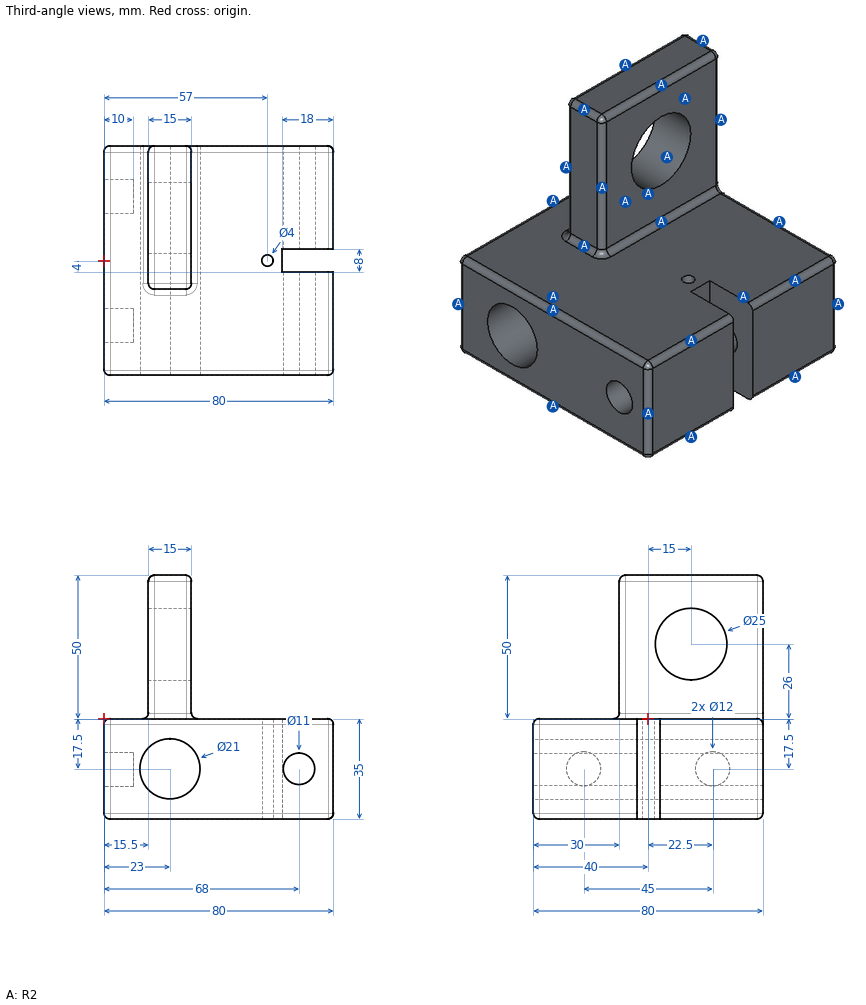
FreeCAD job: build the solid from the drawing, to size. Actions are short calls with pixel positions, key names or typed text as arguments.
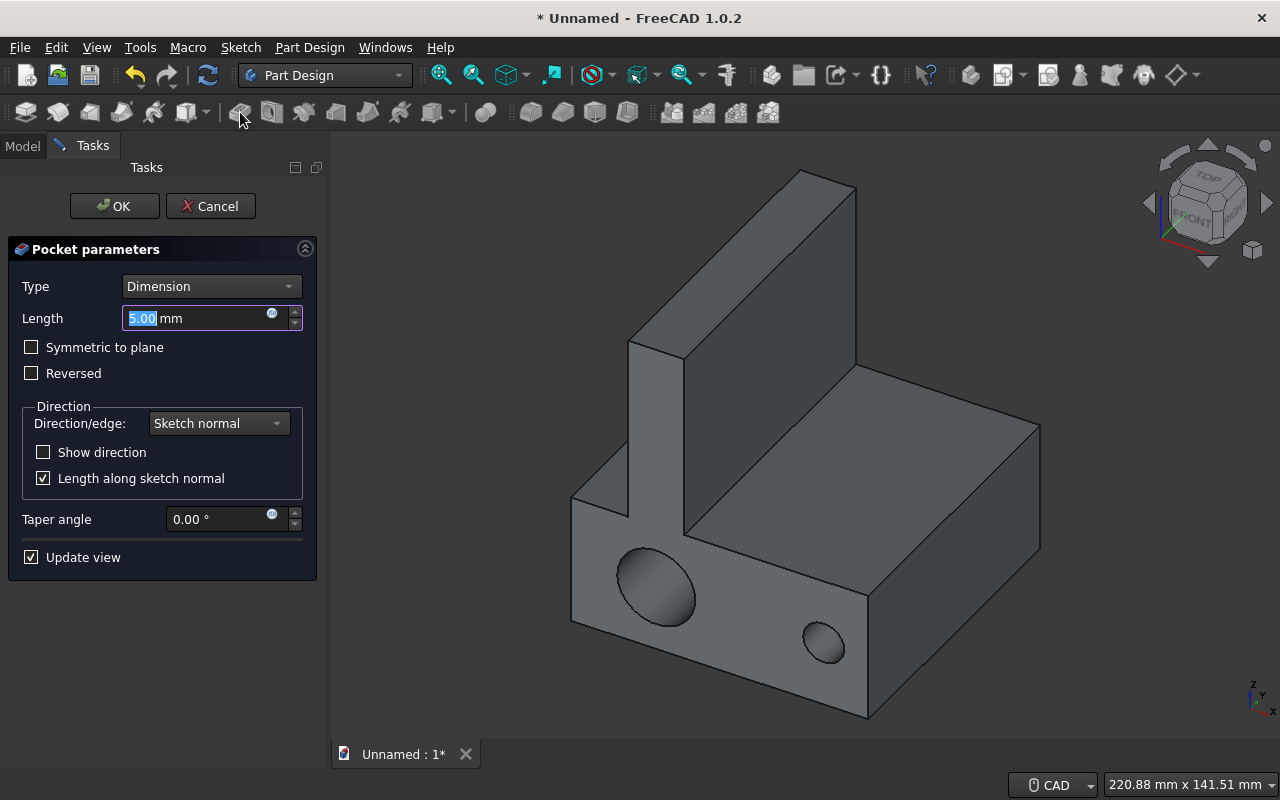
text(10)
key(Tab)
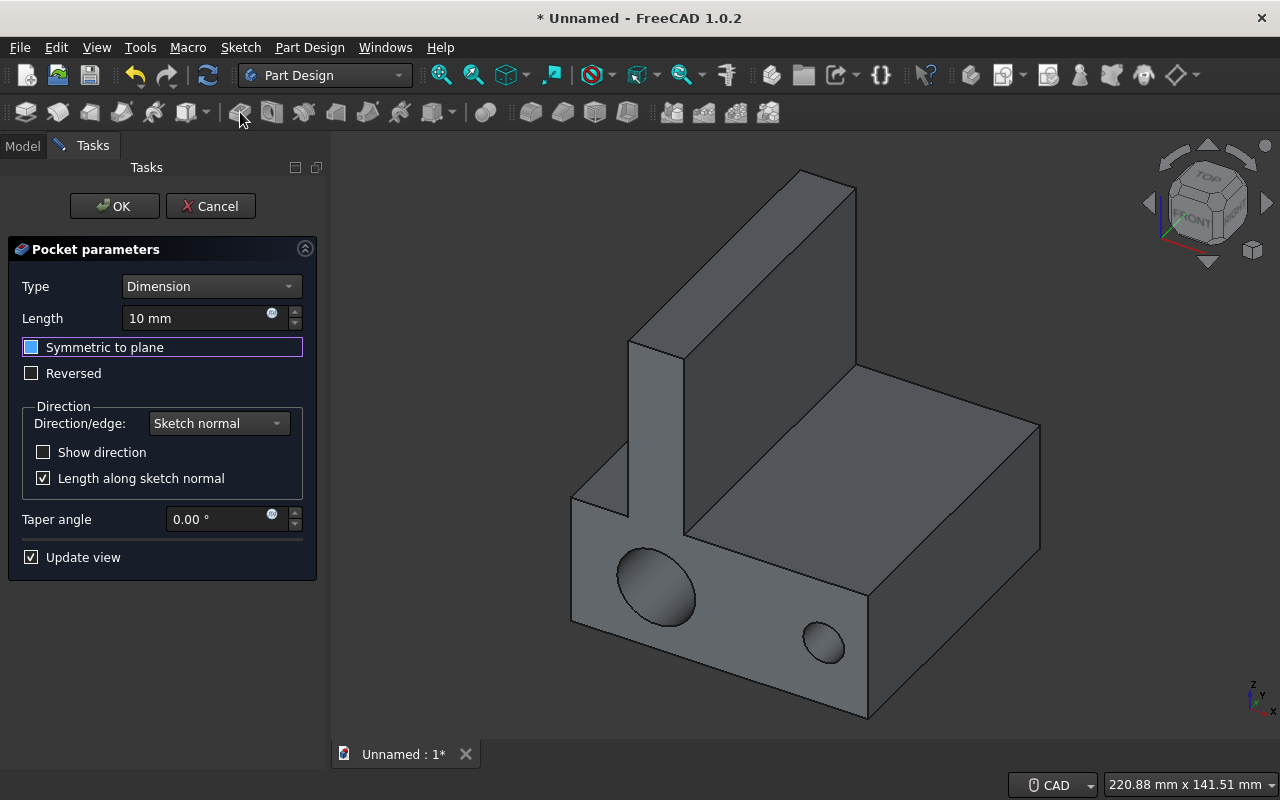
click(30, 373)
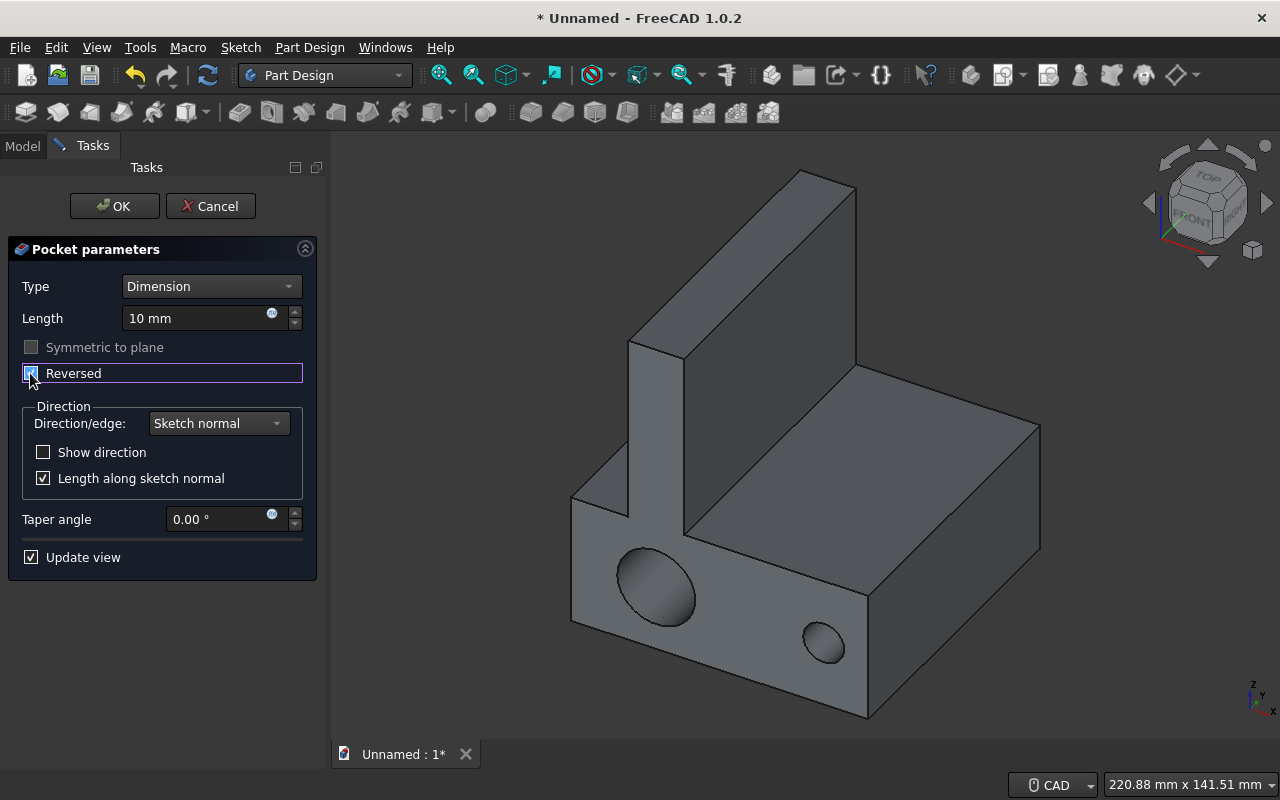
click(115, 206)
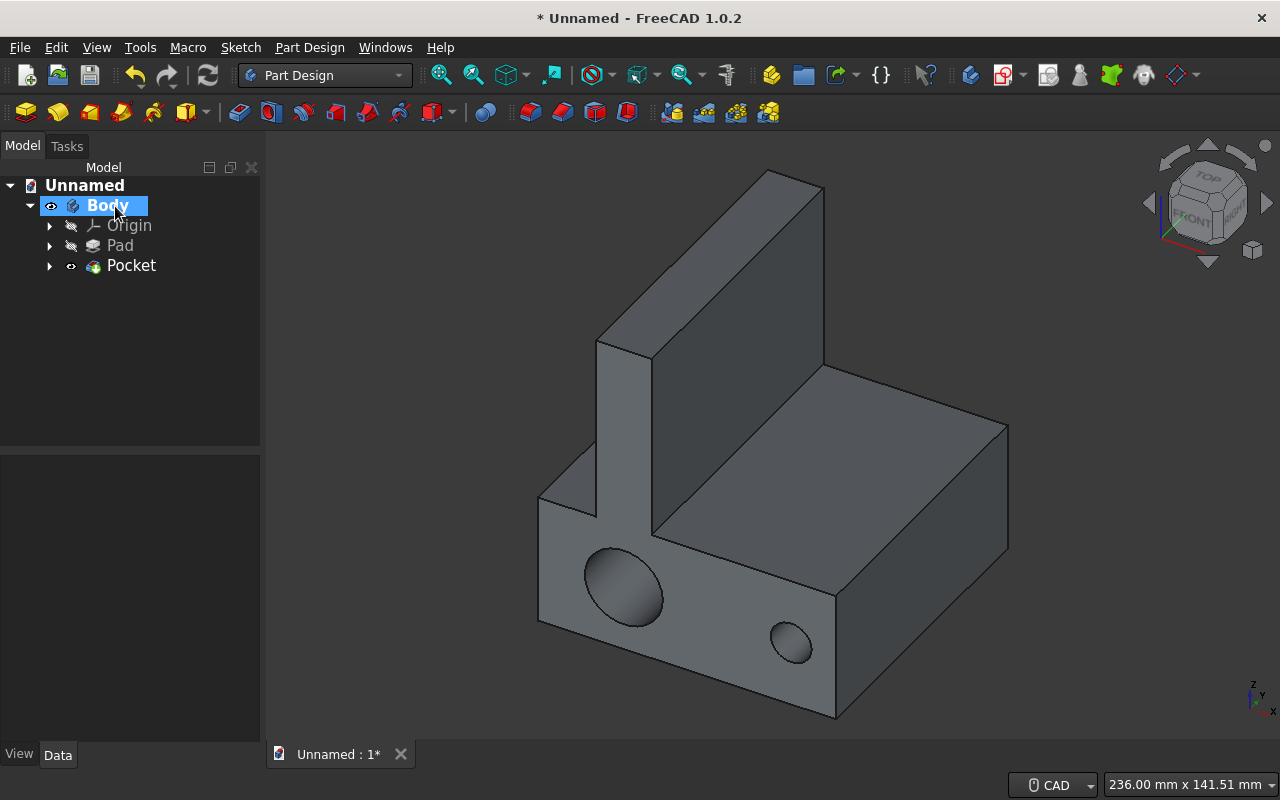
click(762, 336)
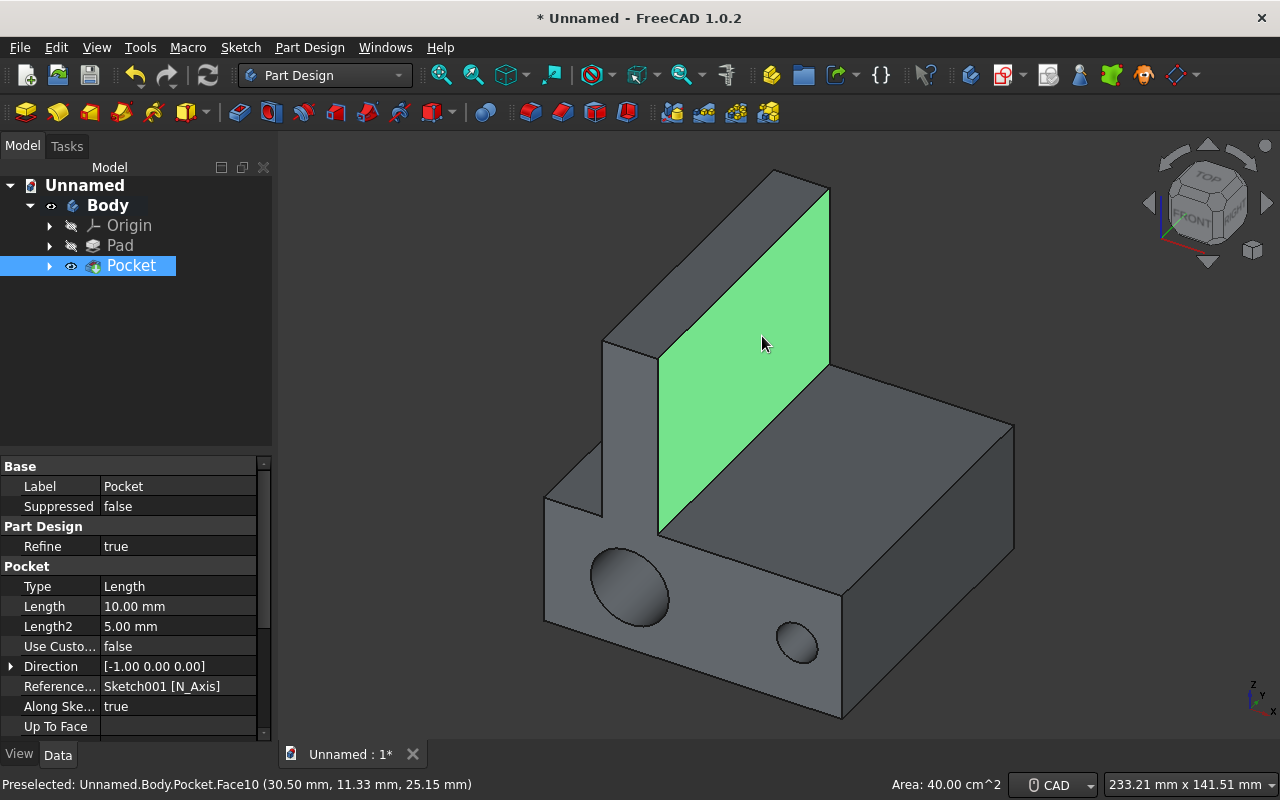
click(1004, 76)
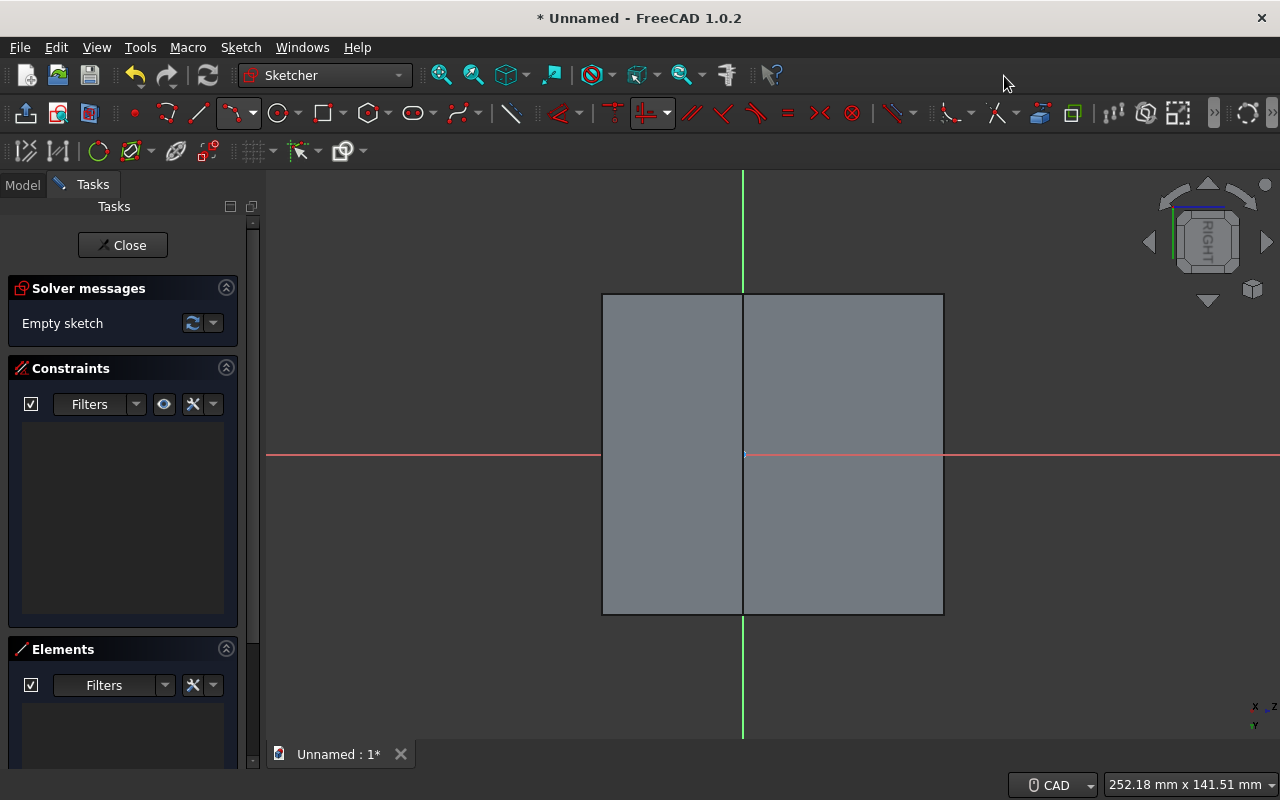
scroll(957, 308, up, 4)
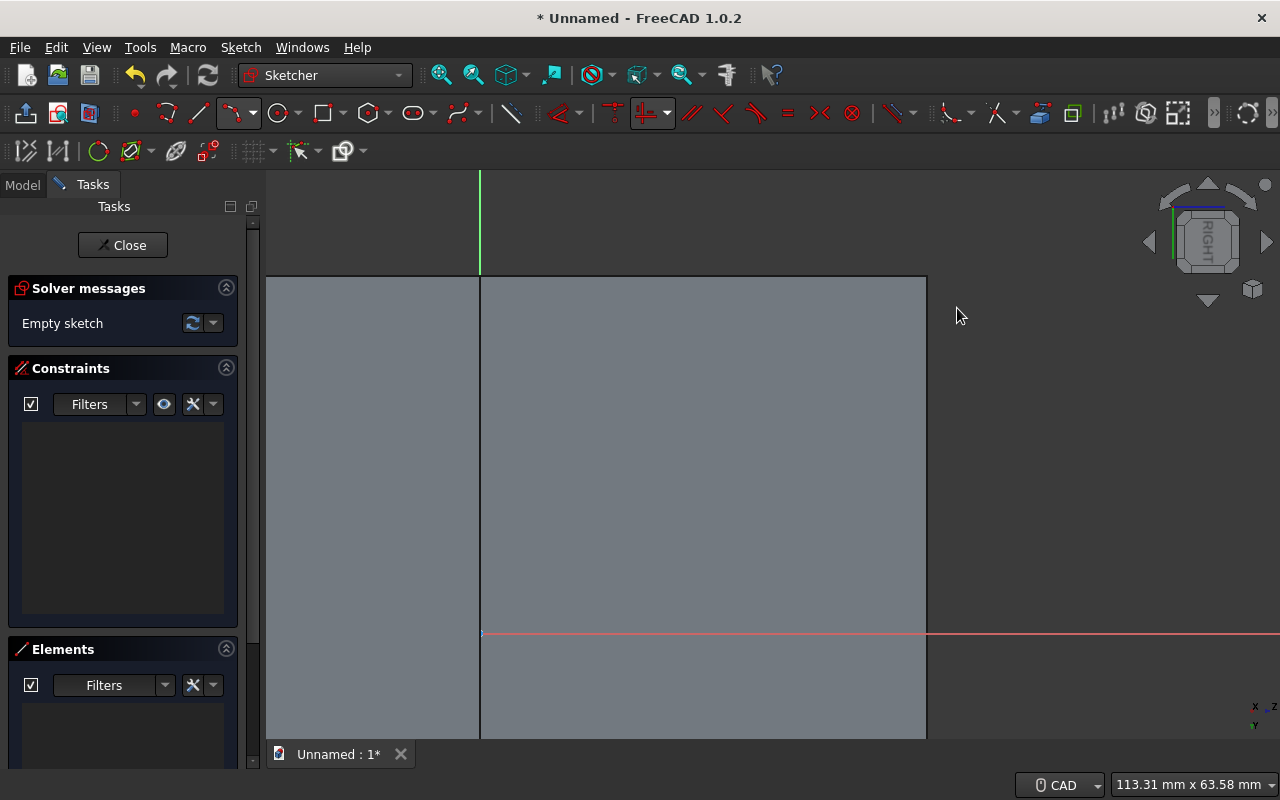
click(324, 114)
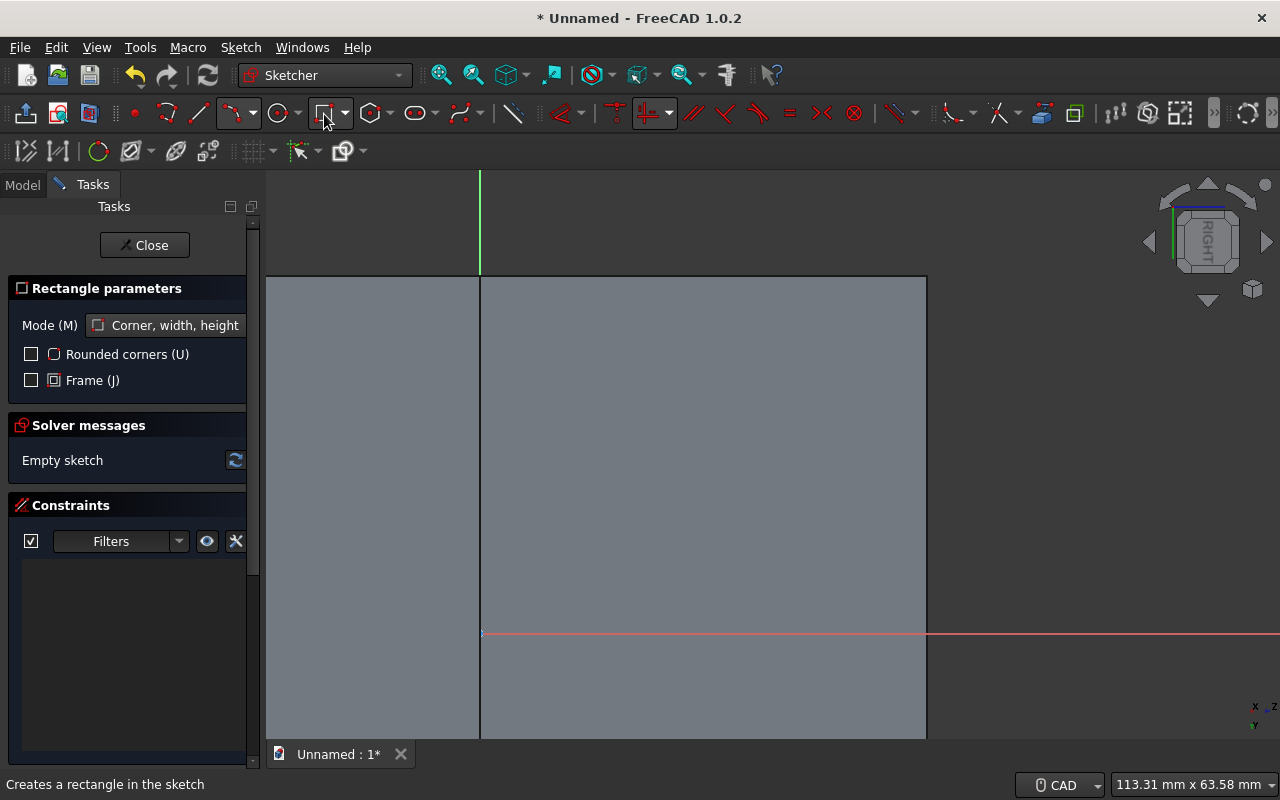
click(480, 276)
click(927, 544)
key(Escape)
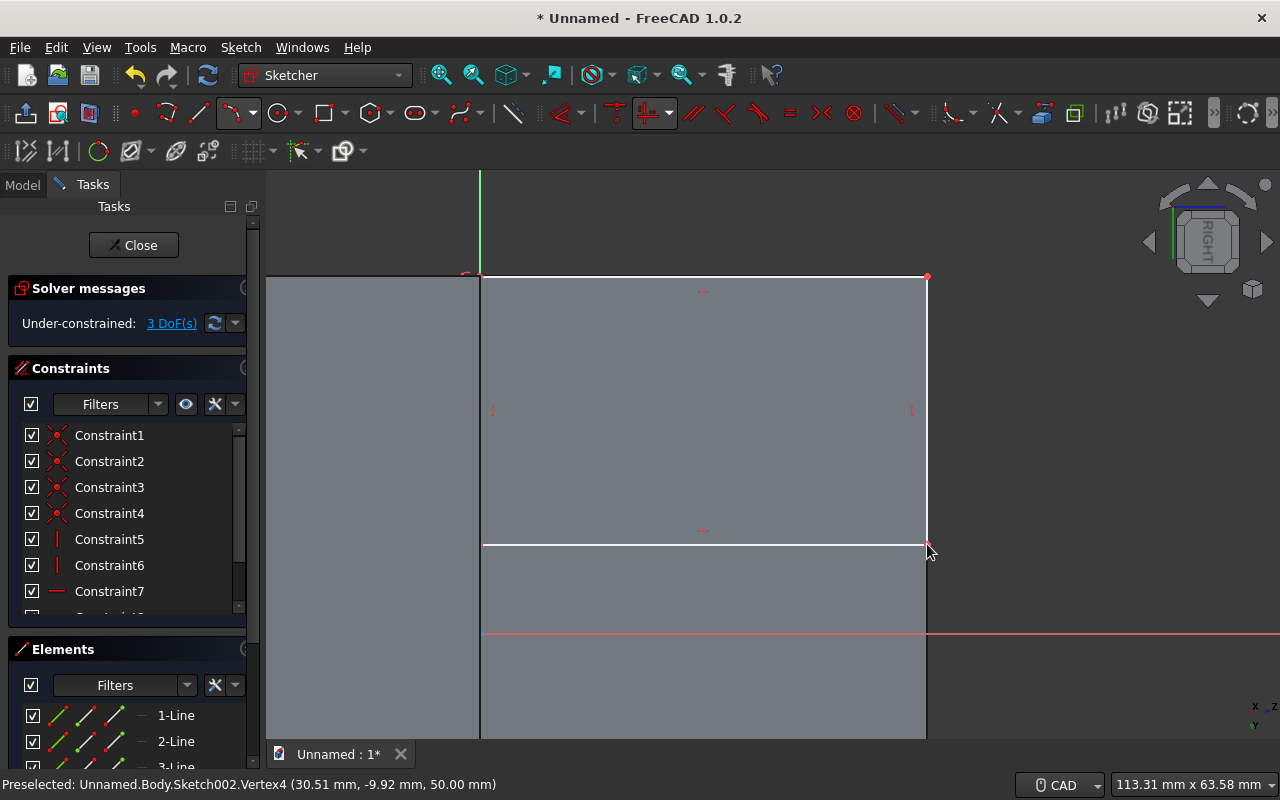
click(560, 114)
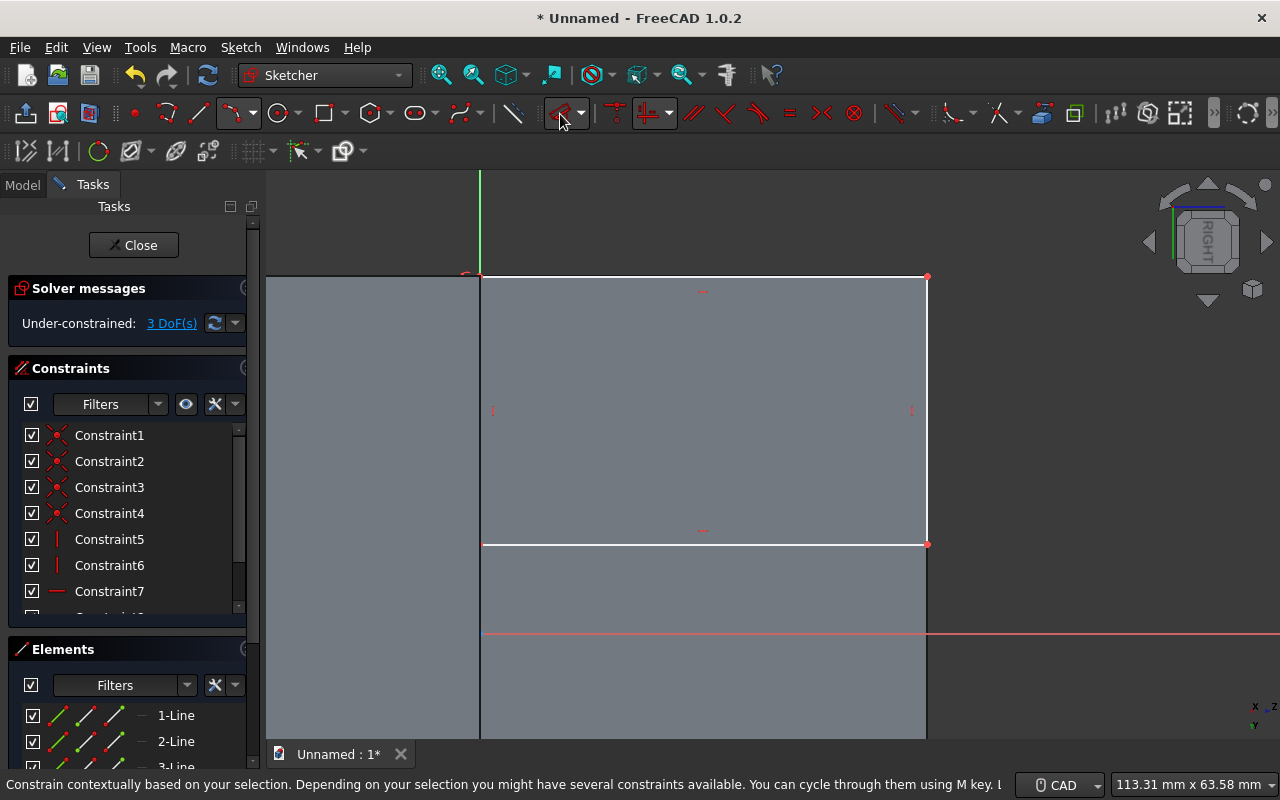
click(480, 357)
click(446, 411)